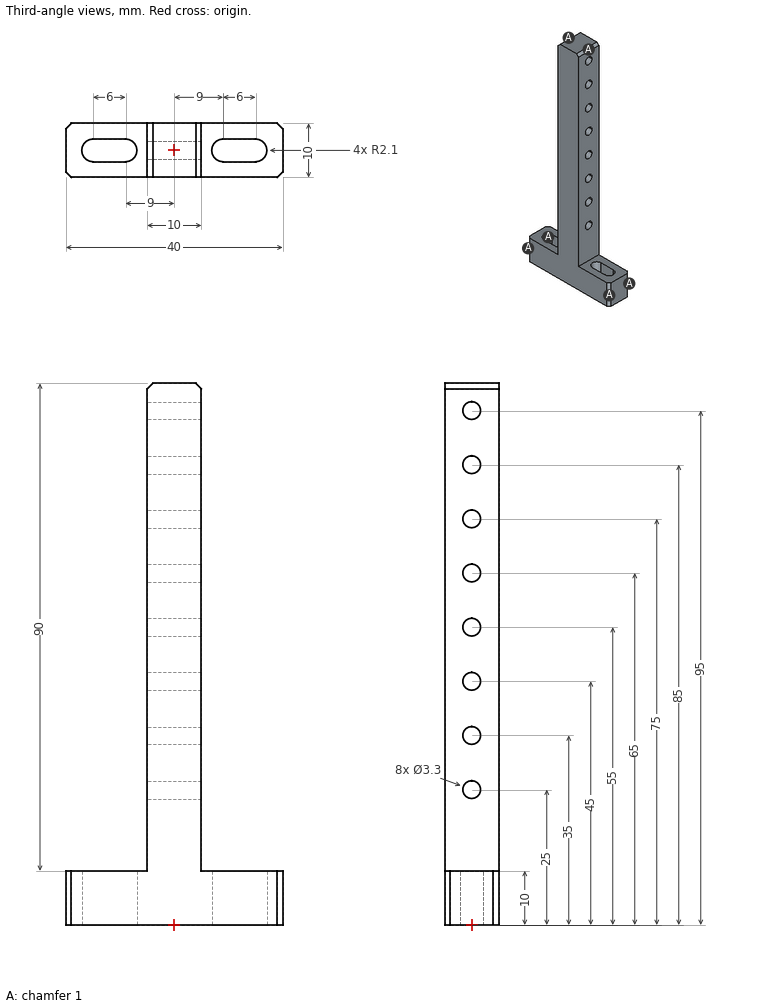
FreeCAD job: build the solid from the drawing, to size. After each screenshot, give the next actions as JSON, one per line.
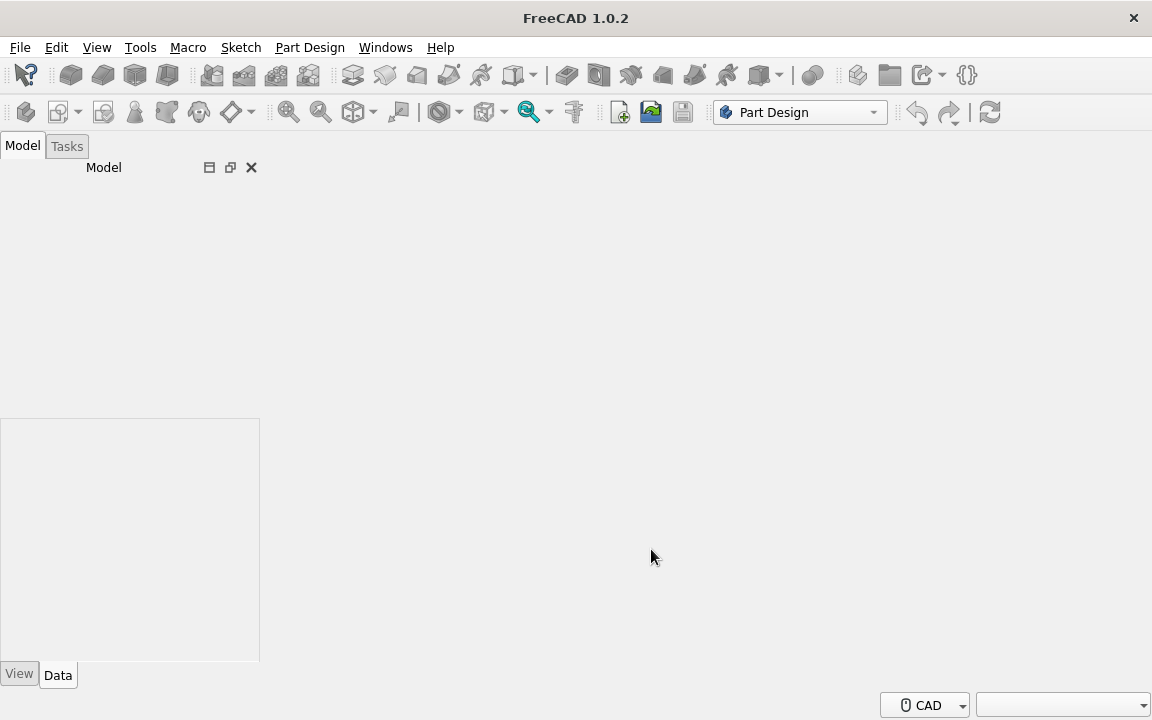
{"action": "left_click", "coordinate": [620, 112]}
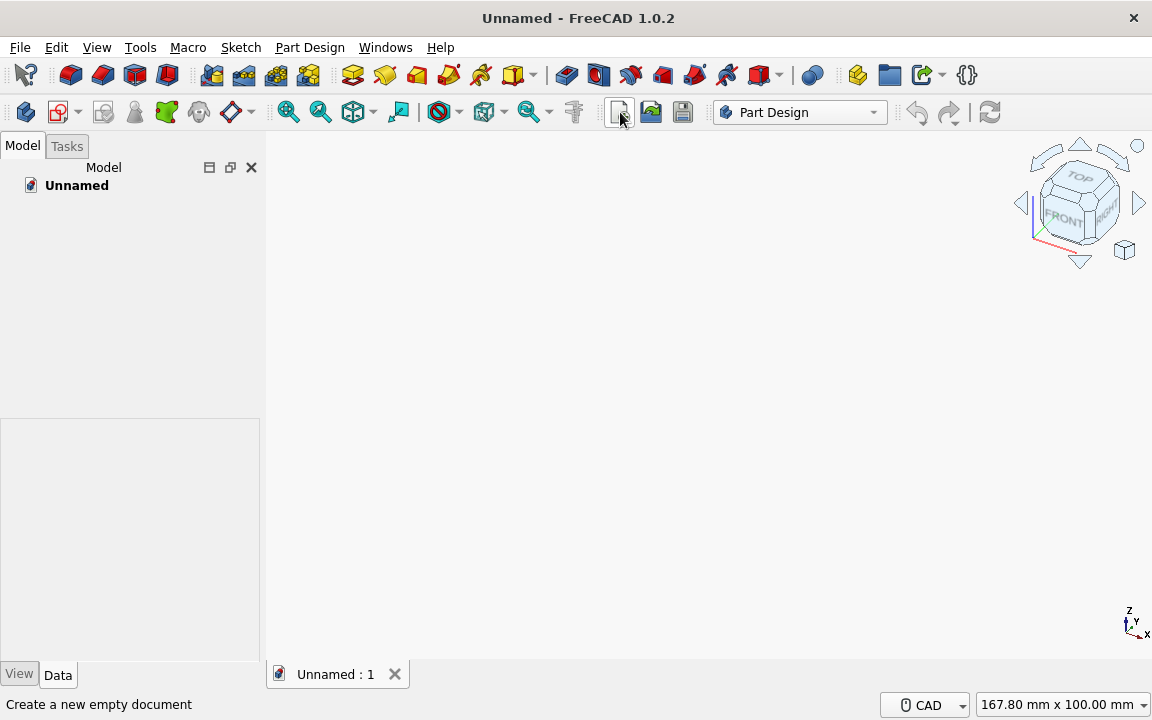
{"action": "left_click", "coordinate": [58, 112]}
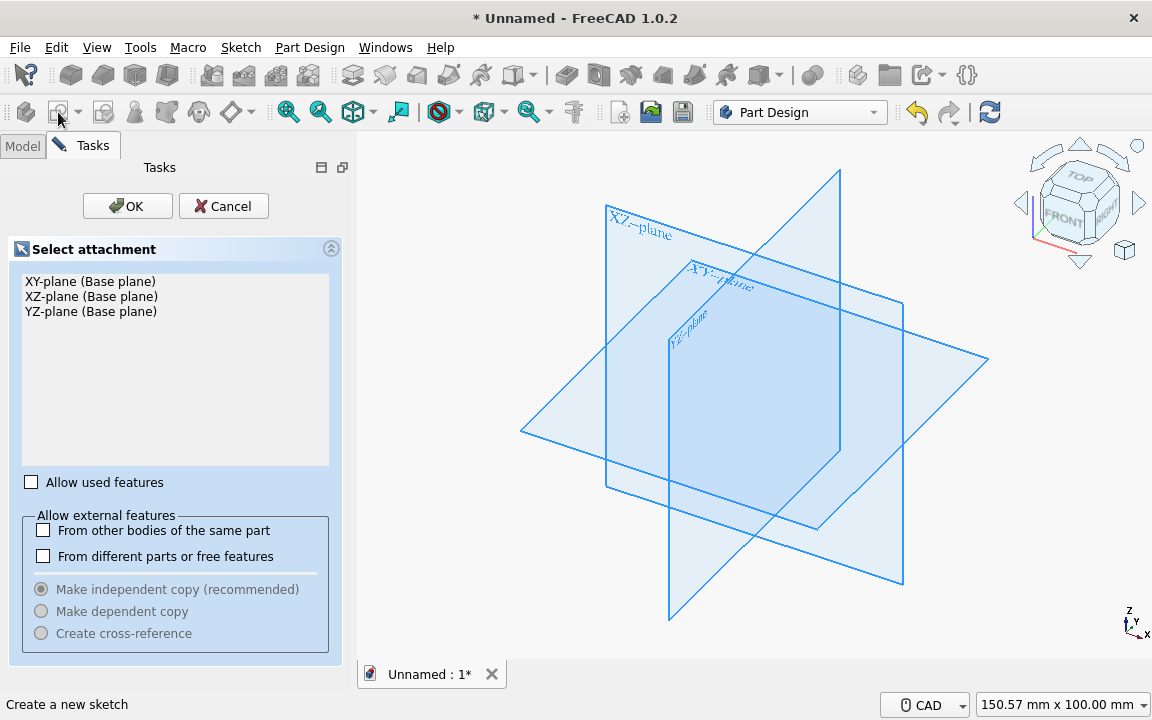
{"action": "left_click", "coordinate": [82, 282]}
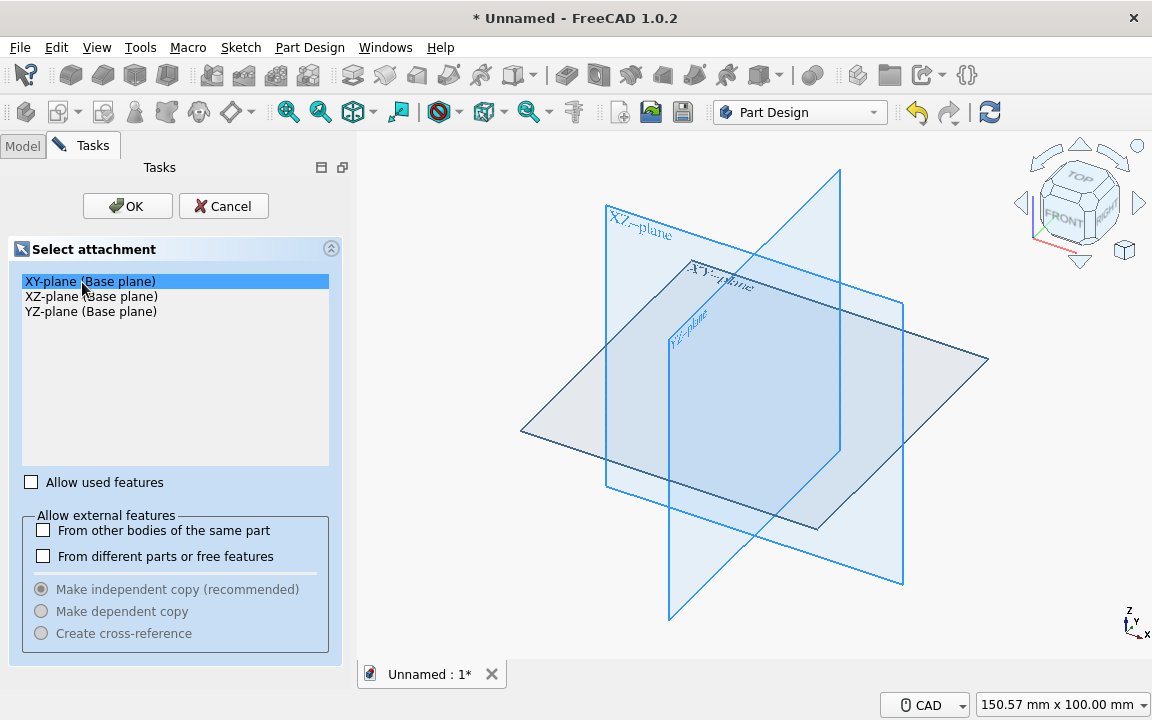
{"action": "left_click", "coordinate": [128, 206]}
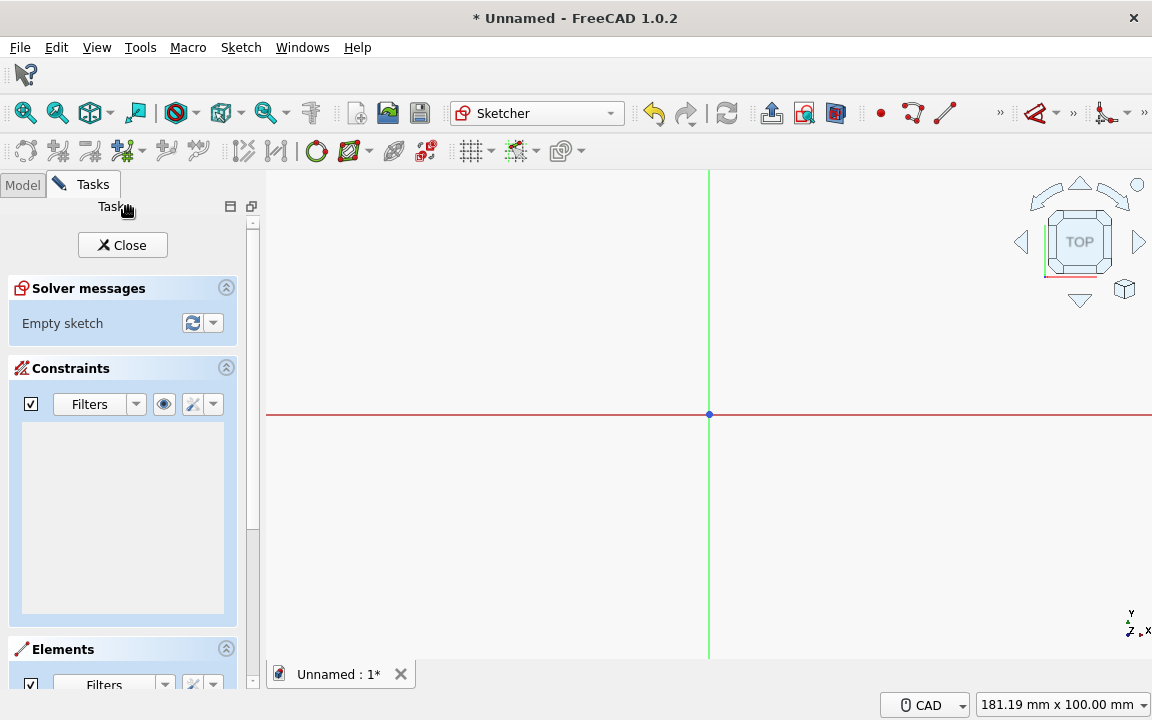
{"action": "scroll", "coordinate": [749, 415], "scroll_direction": "up", "scroll_amount": 5}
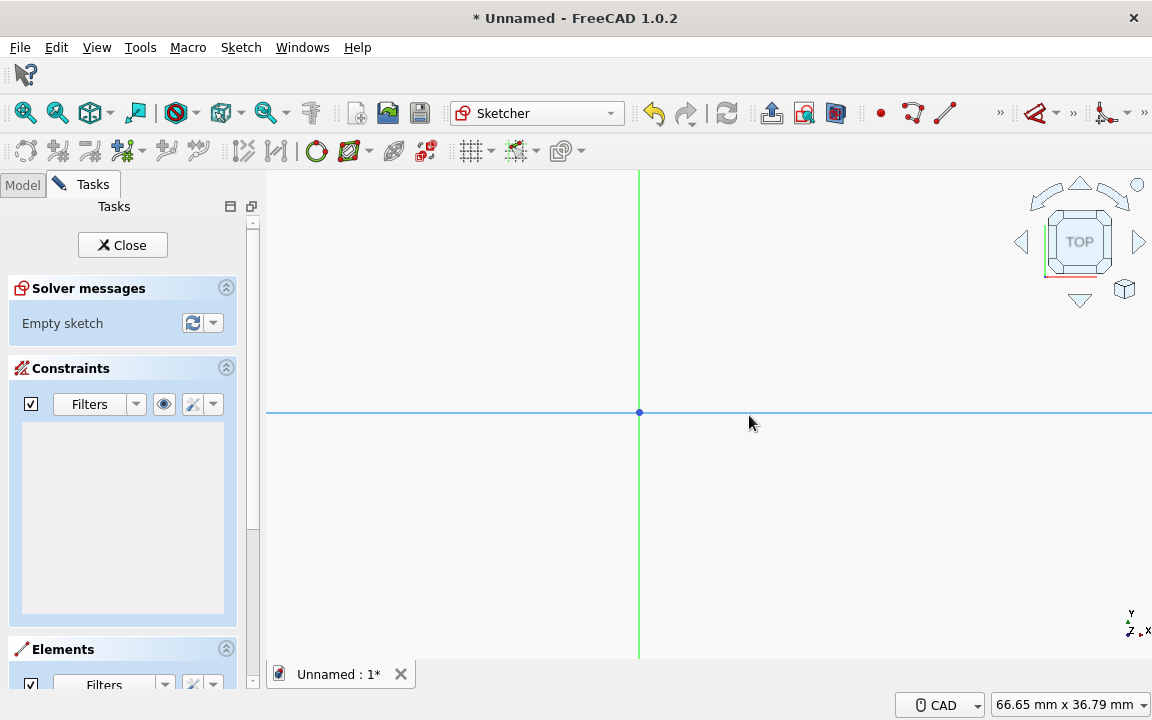
{"action": "key", "text": "g v"}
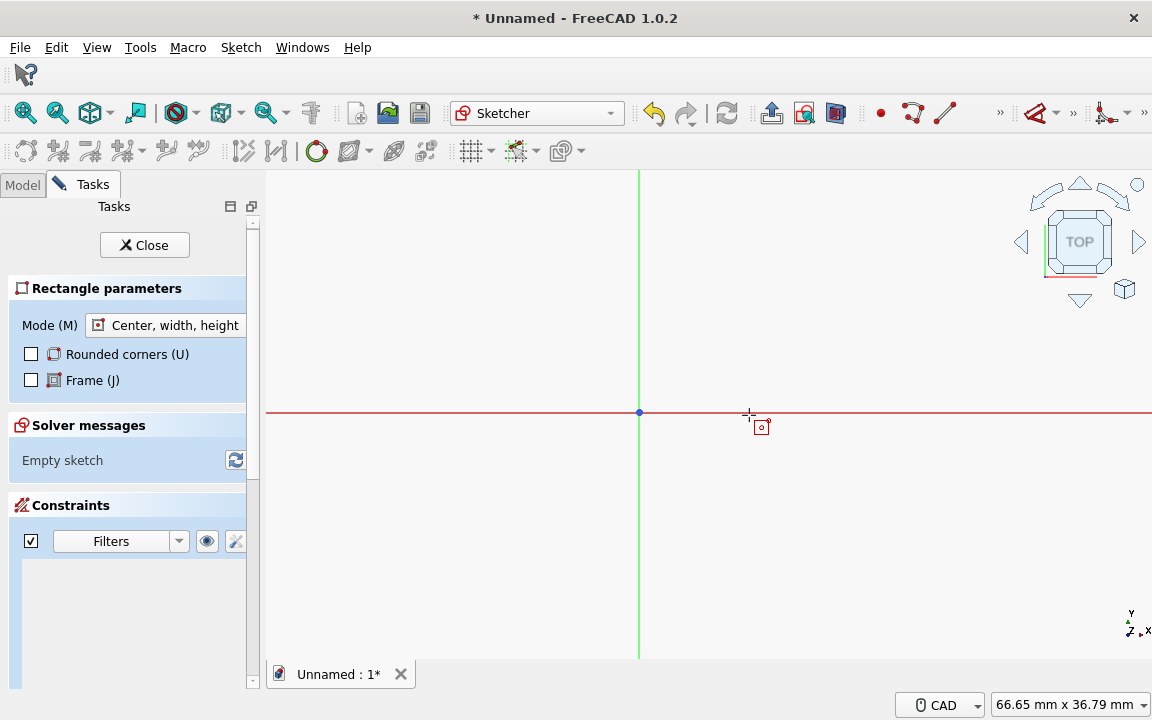
{"action": "left_click", "coordinate": [639, 413]}
{"action": "mouse_move", "coordinate": [905, 346]}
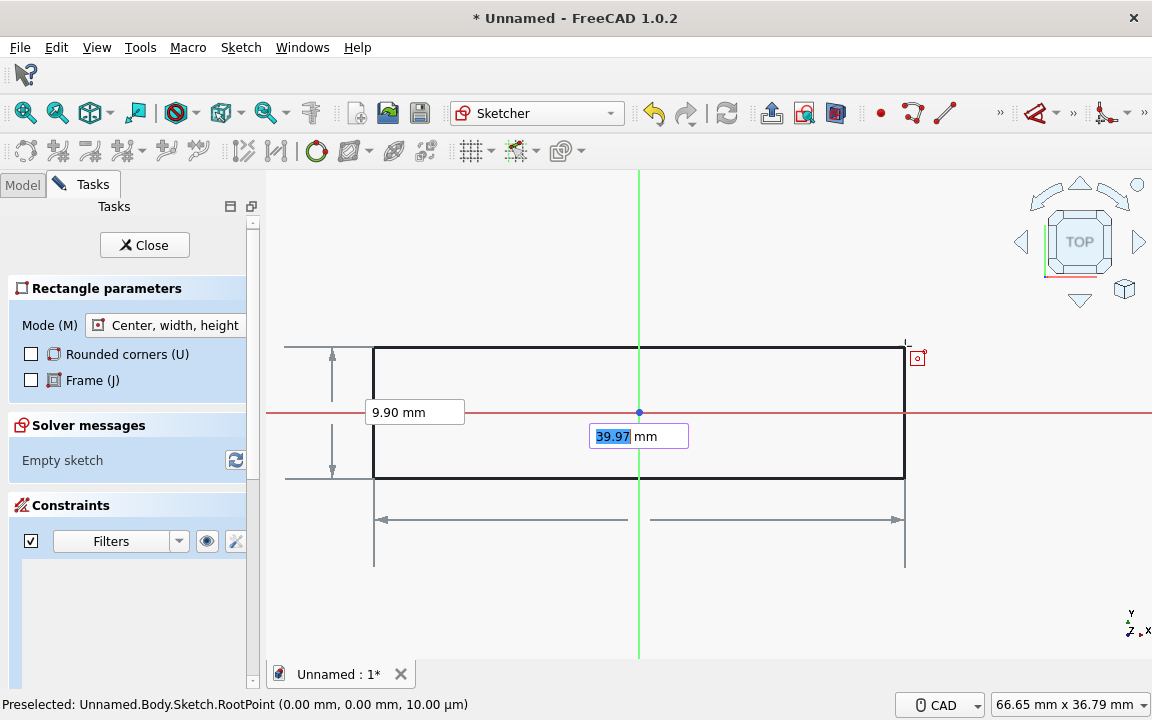
{"action": "type", "text": "40"}
{"action": "key", "text": "Tab"}
{"action": "type", "text": "10"}
{"action": "key", "text": "Return"}
{"action": "key", "text": "Escape"}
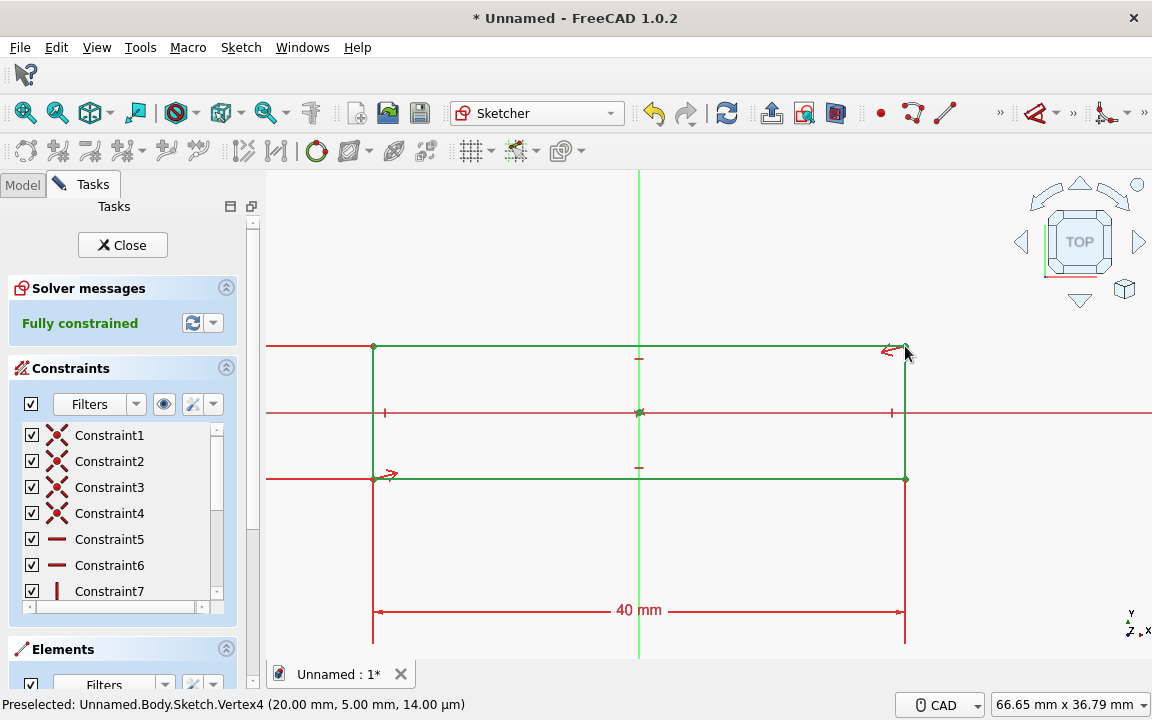
{"action": "left_click", "coordinate": [123, 245]}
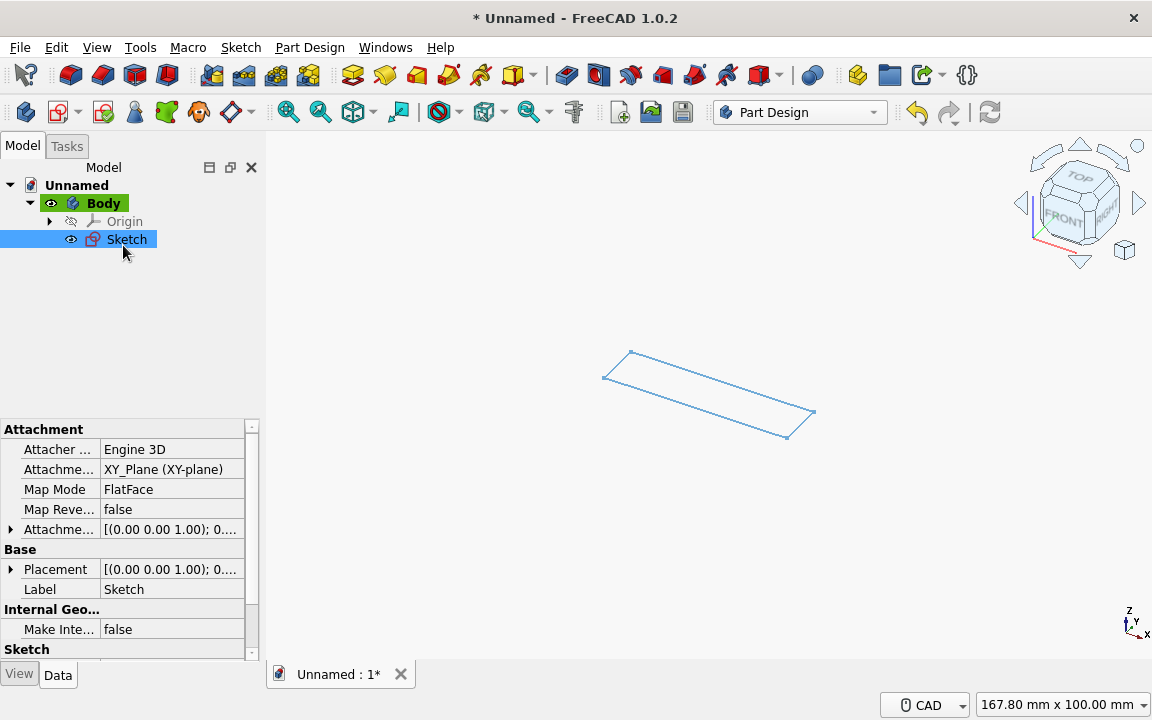
{"action": "left_click", "coordinate": [354, 76]}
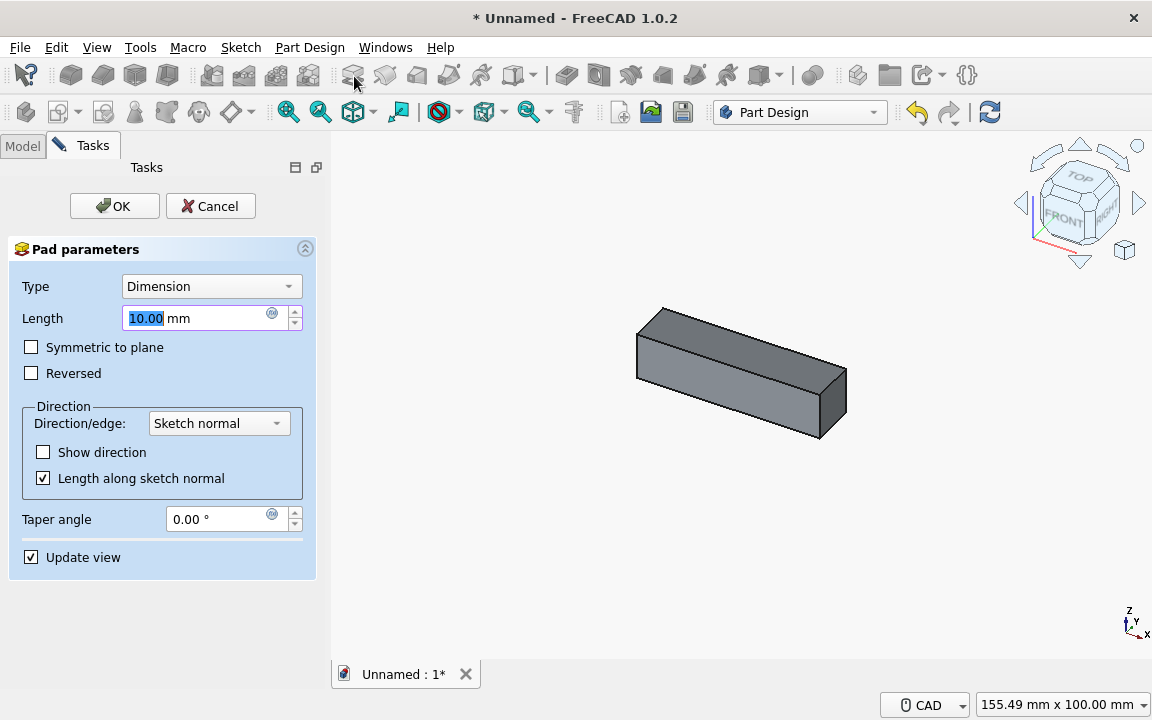
{"action": "type", "text": "10"}
{"action": "key", "text": "Tab"}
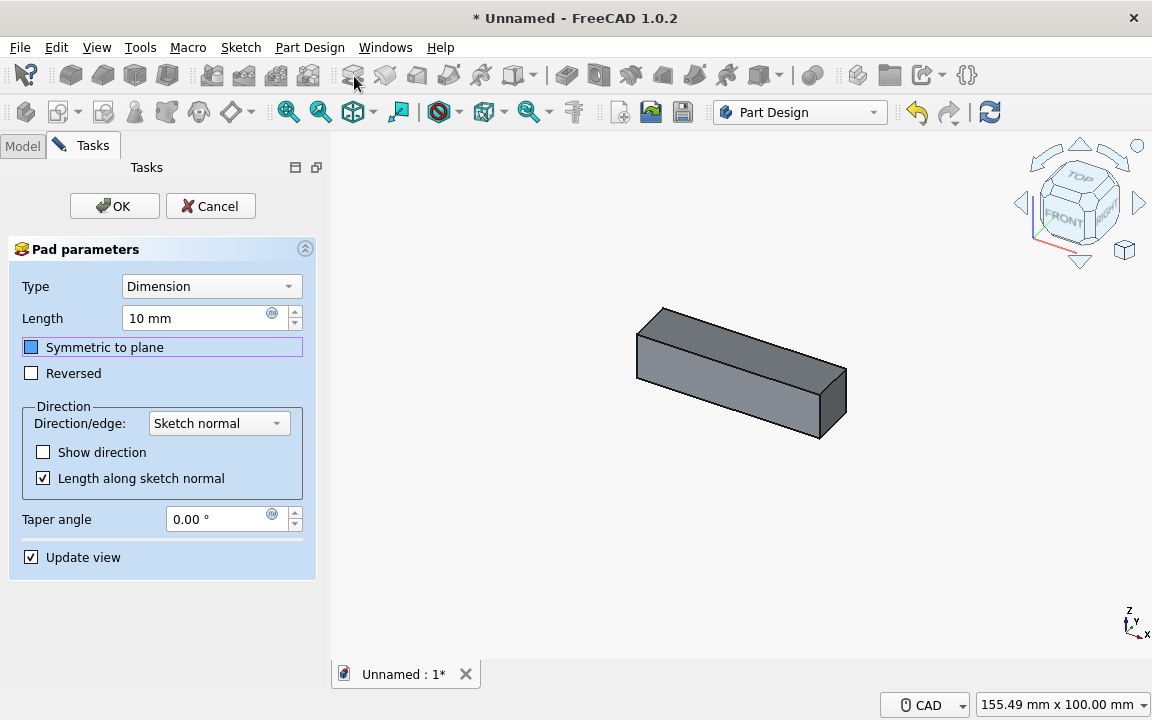
{"action": "left_click", "coordinate": [115, 206]}